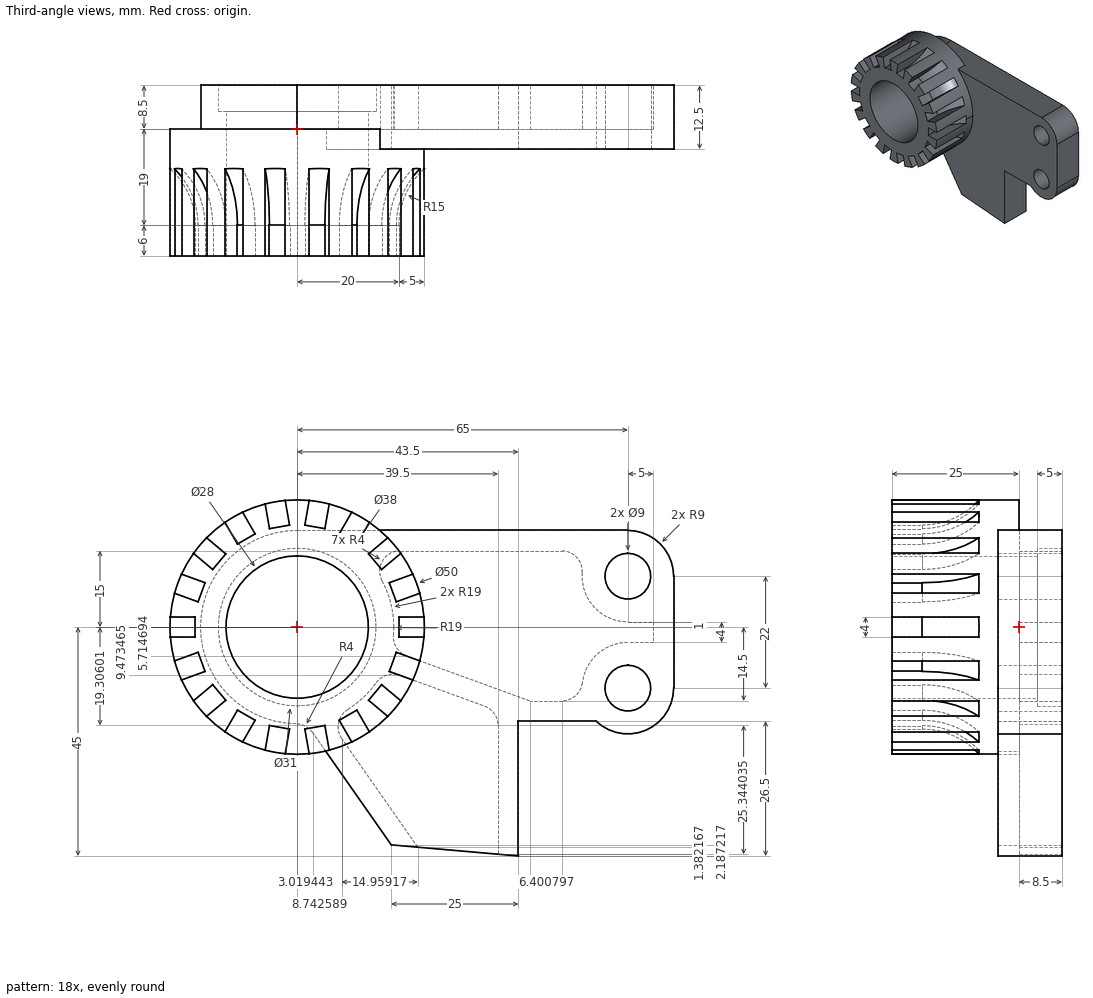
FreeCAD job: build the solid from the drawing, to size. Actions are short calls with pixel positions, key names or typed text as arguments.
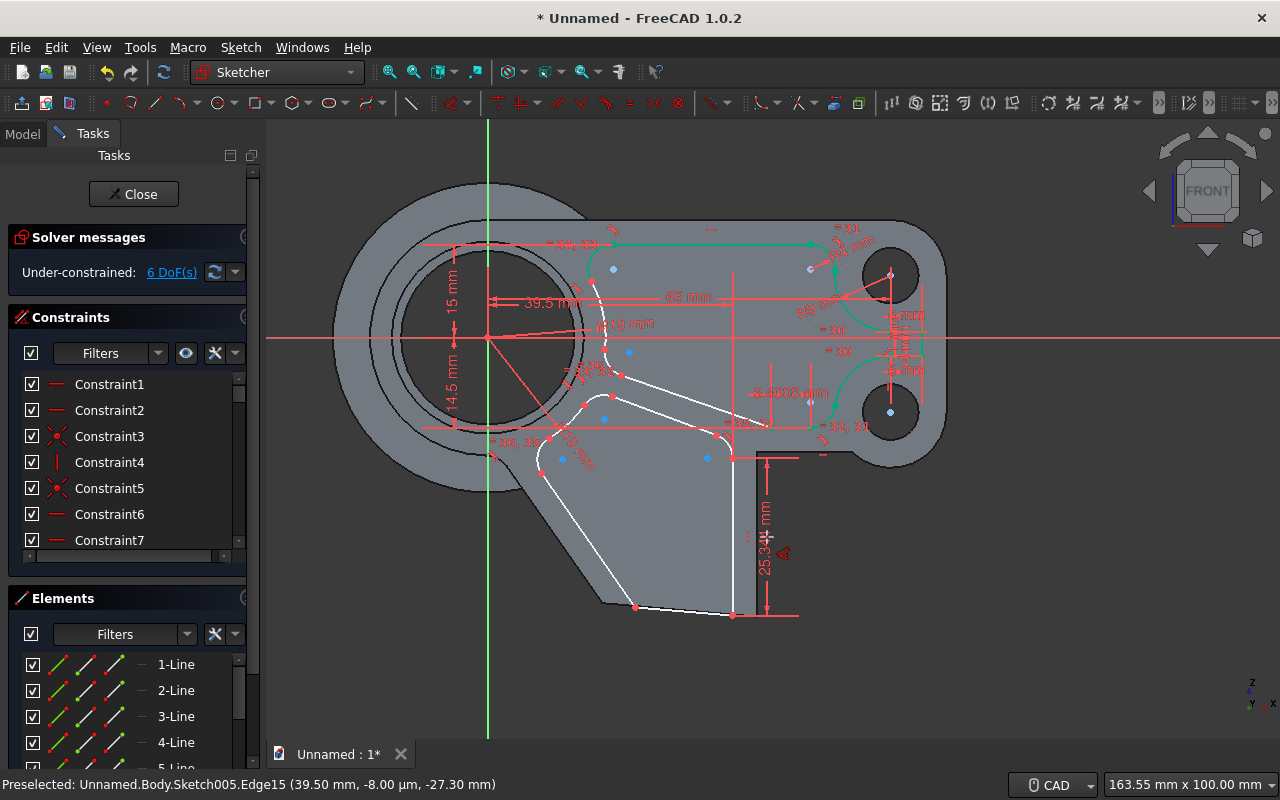
click(621, 375)
click(454, 357)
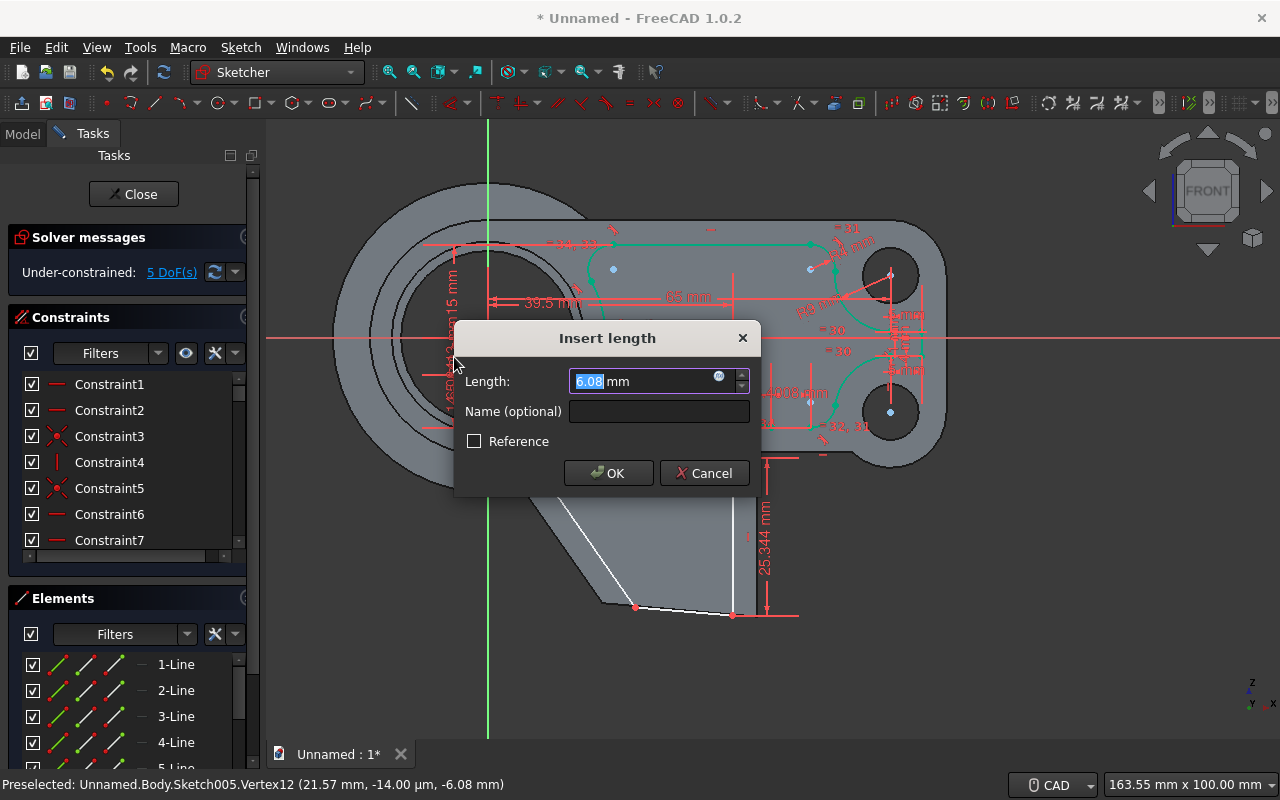
text(5.714694)
key(Return)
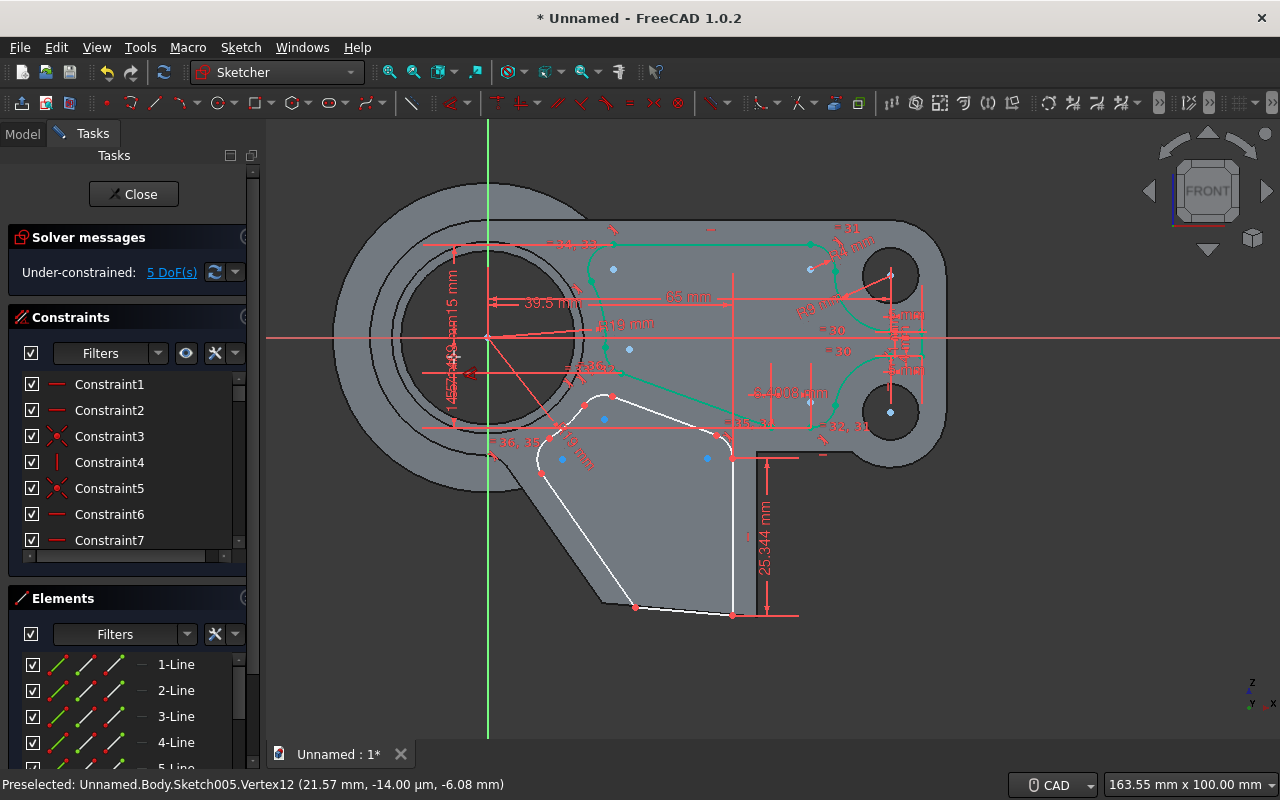
click(613, 397)
click(647, 367)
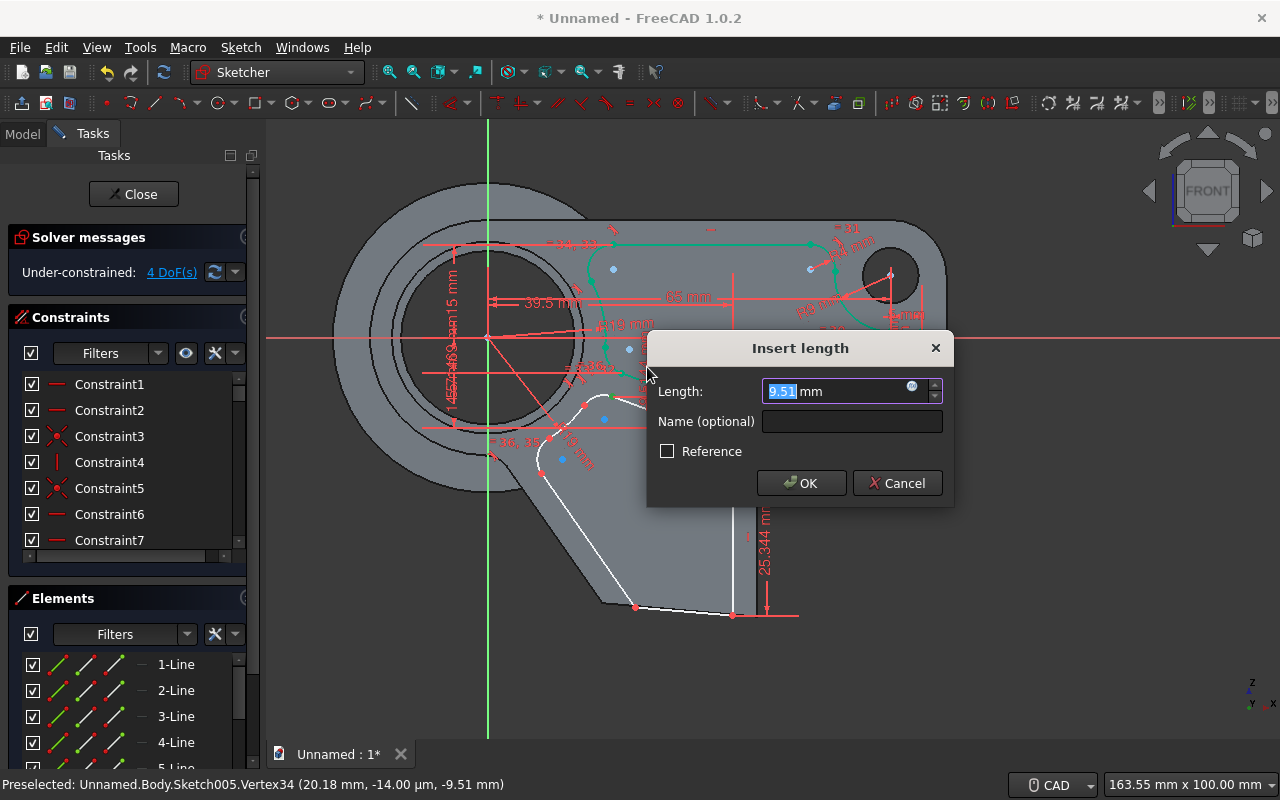
text(9.473465)
key(Return)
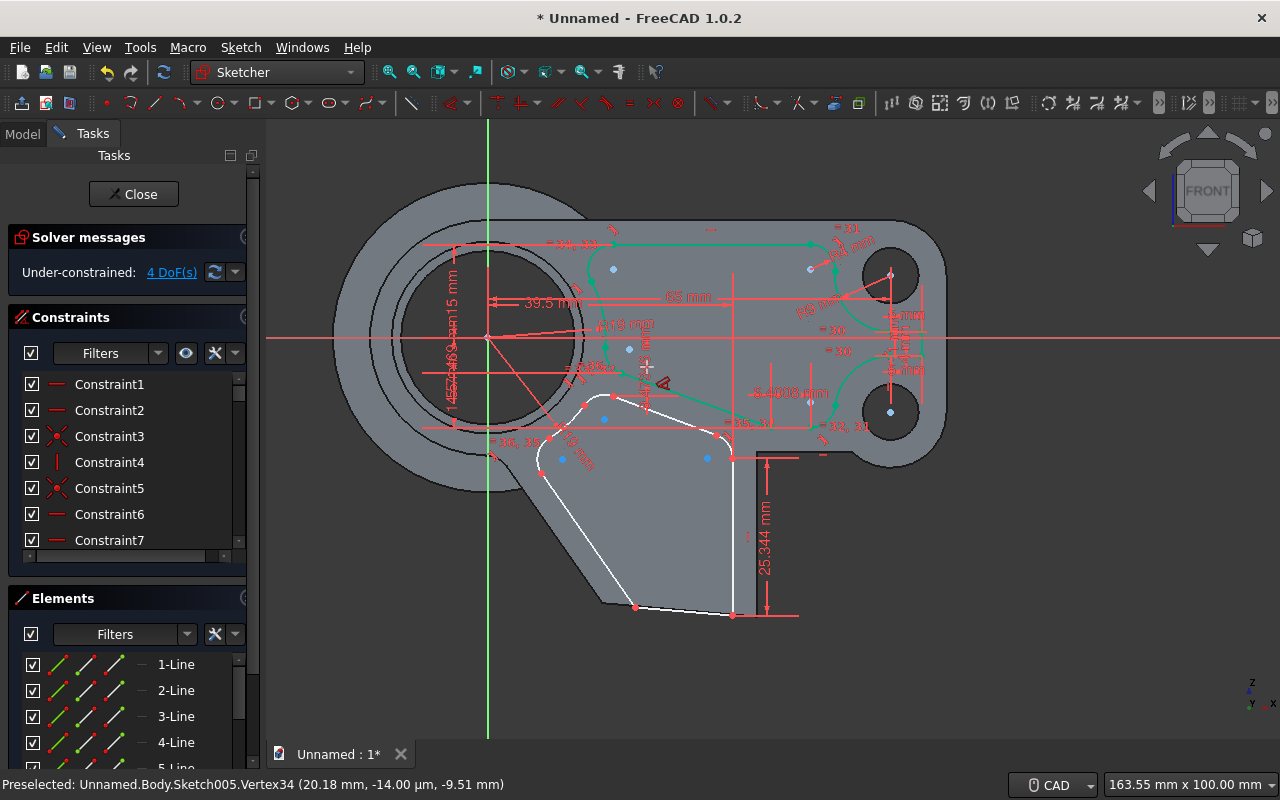
click(733, 458)
click(454, 426)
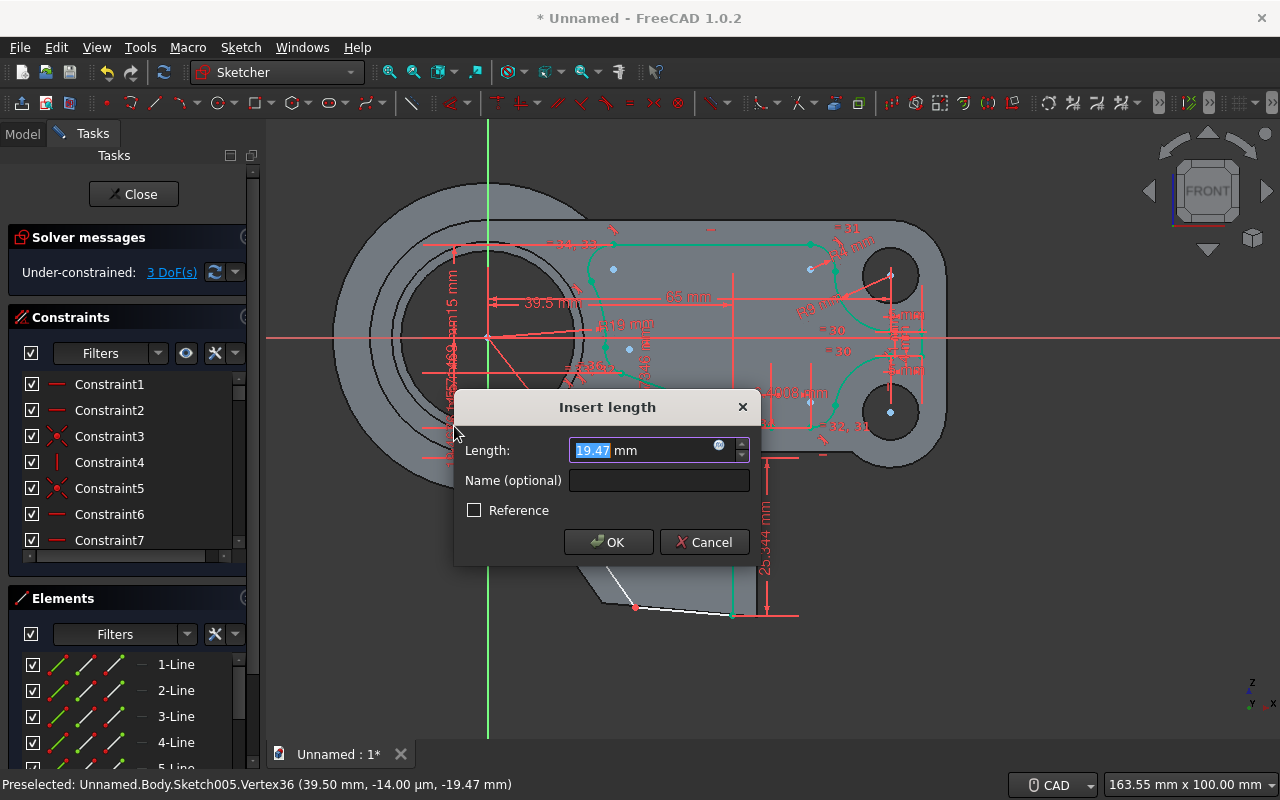
text(19.30601)
key(Return)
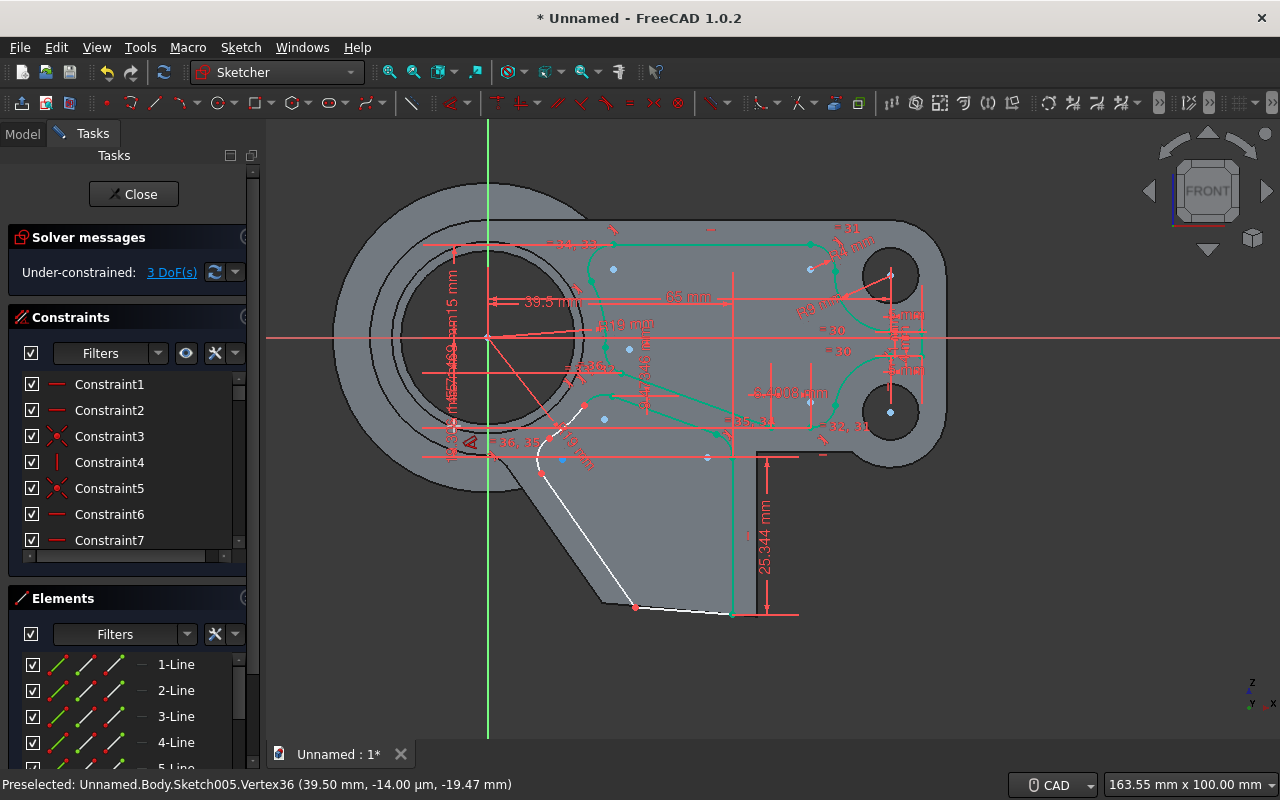
click(542, 474)
click(515, 508)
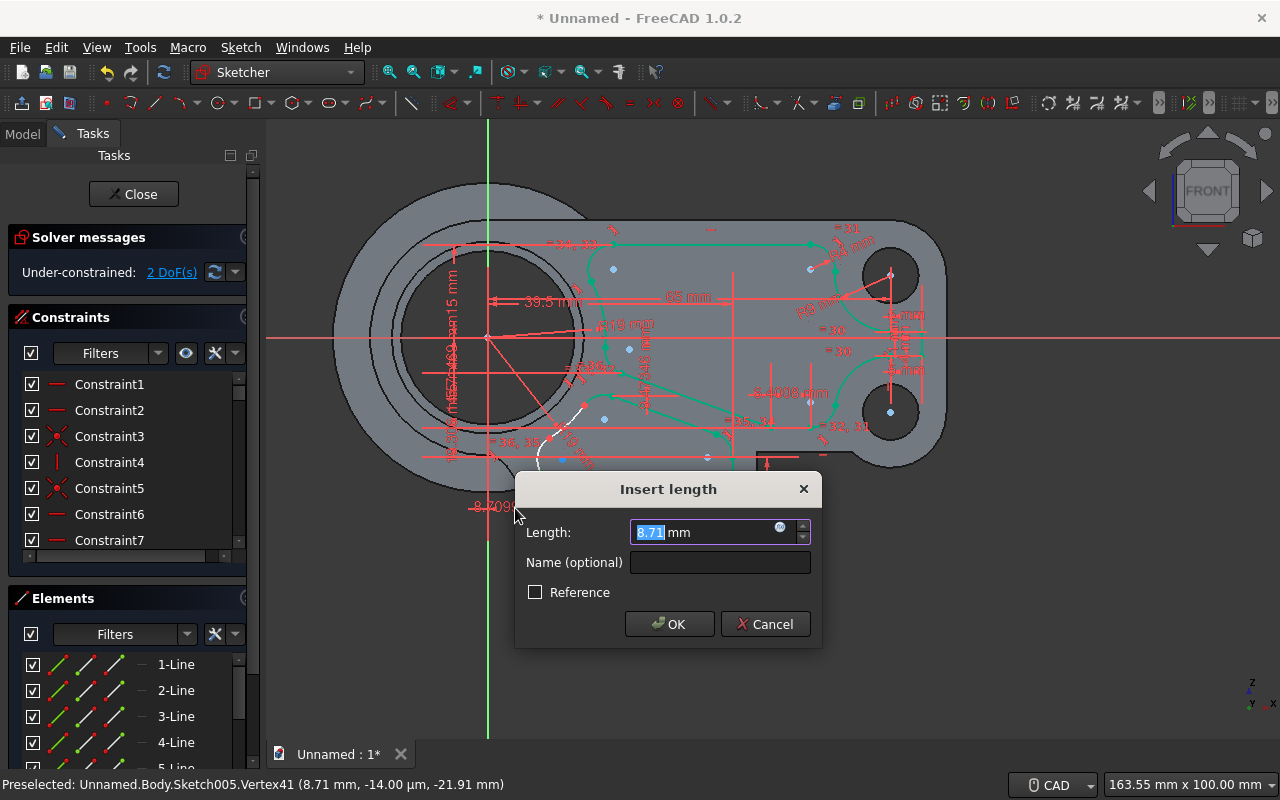
text(8.742589)
key(Return)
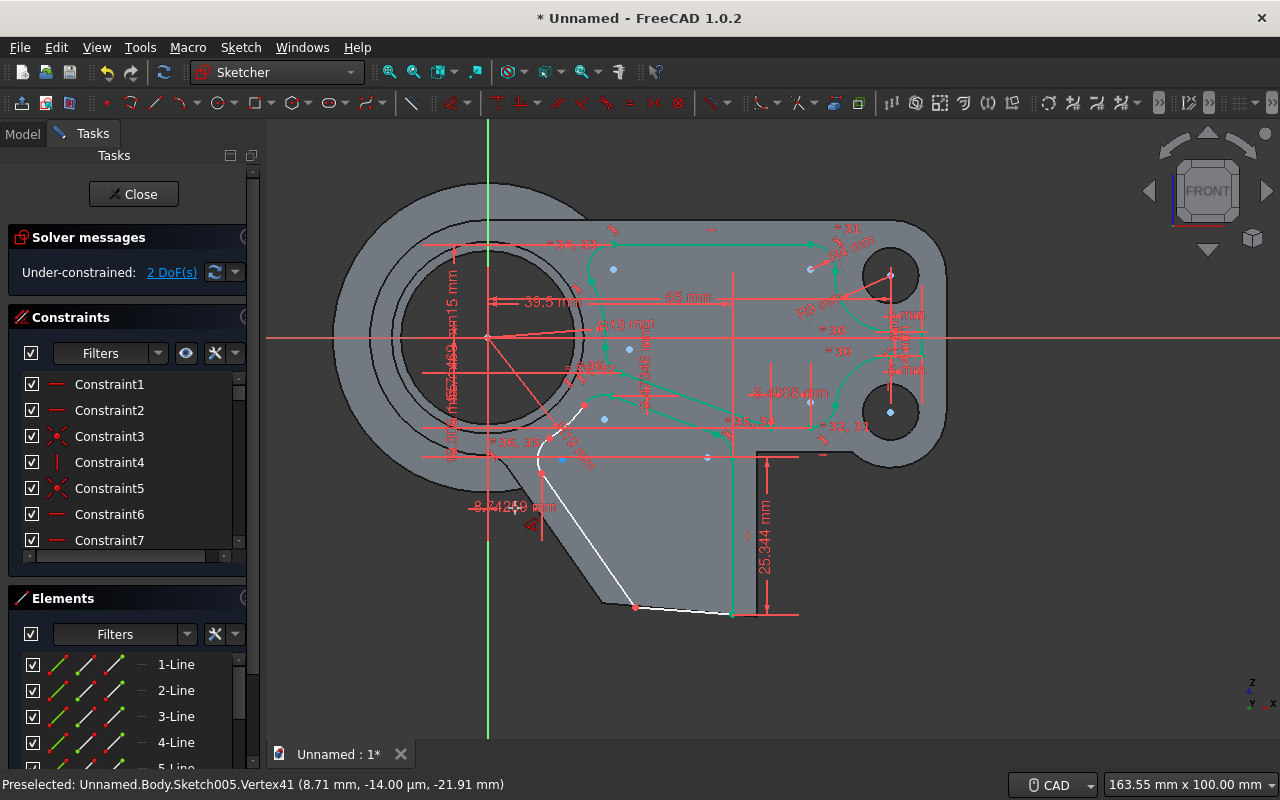
scroll(703, 612, up, 8)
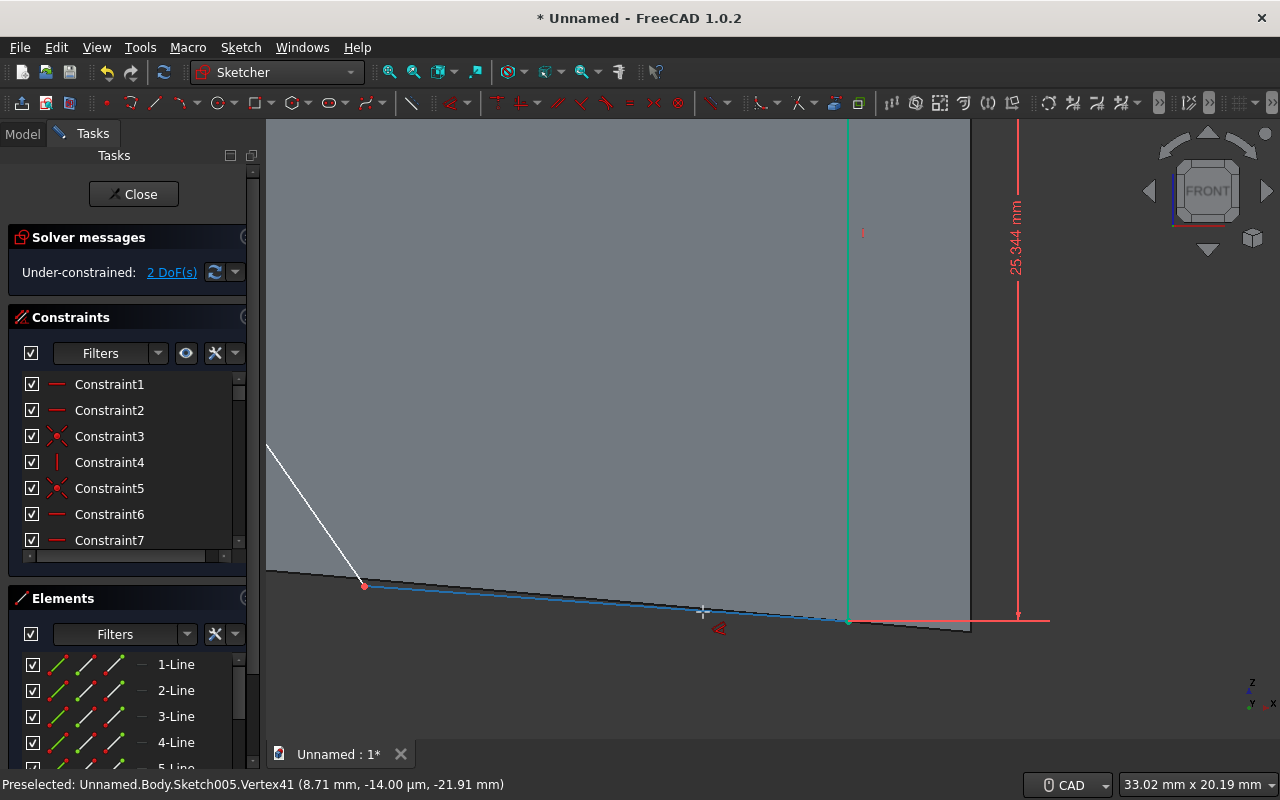
click(703, 611)
click(331, 604)